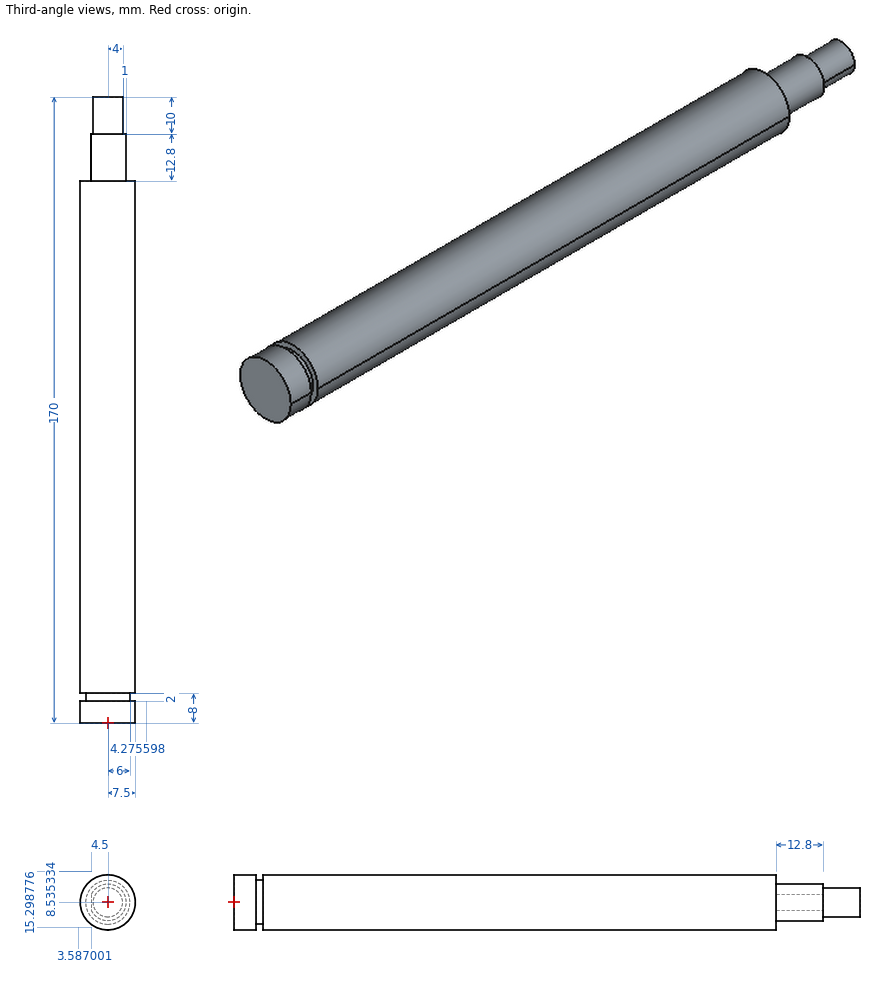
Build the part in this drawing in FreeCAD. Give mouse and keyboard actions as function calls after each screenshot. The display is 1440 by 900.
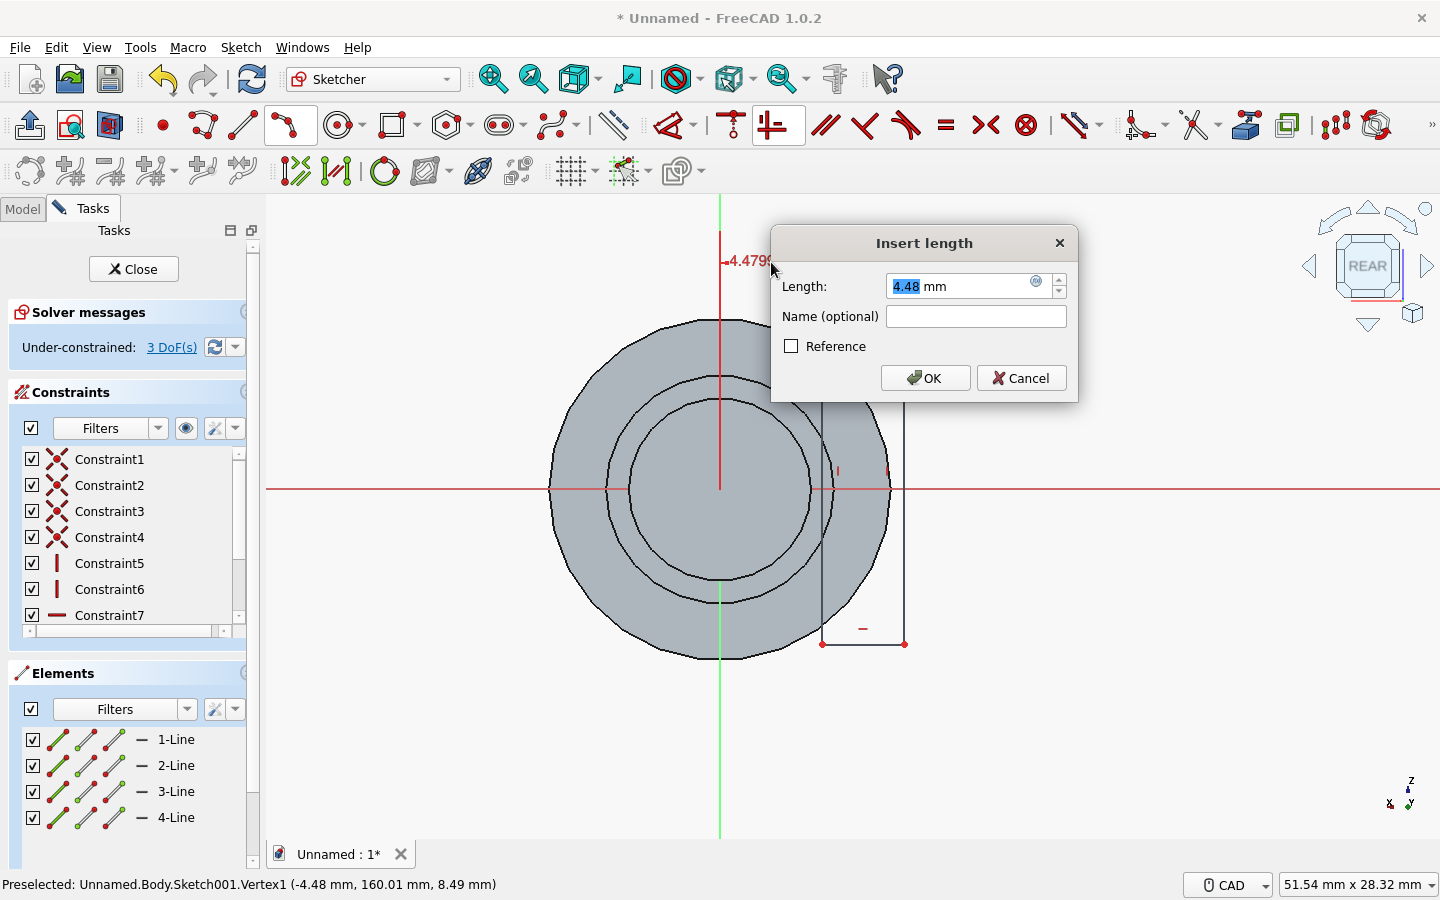
text(4.5)
key(Return)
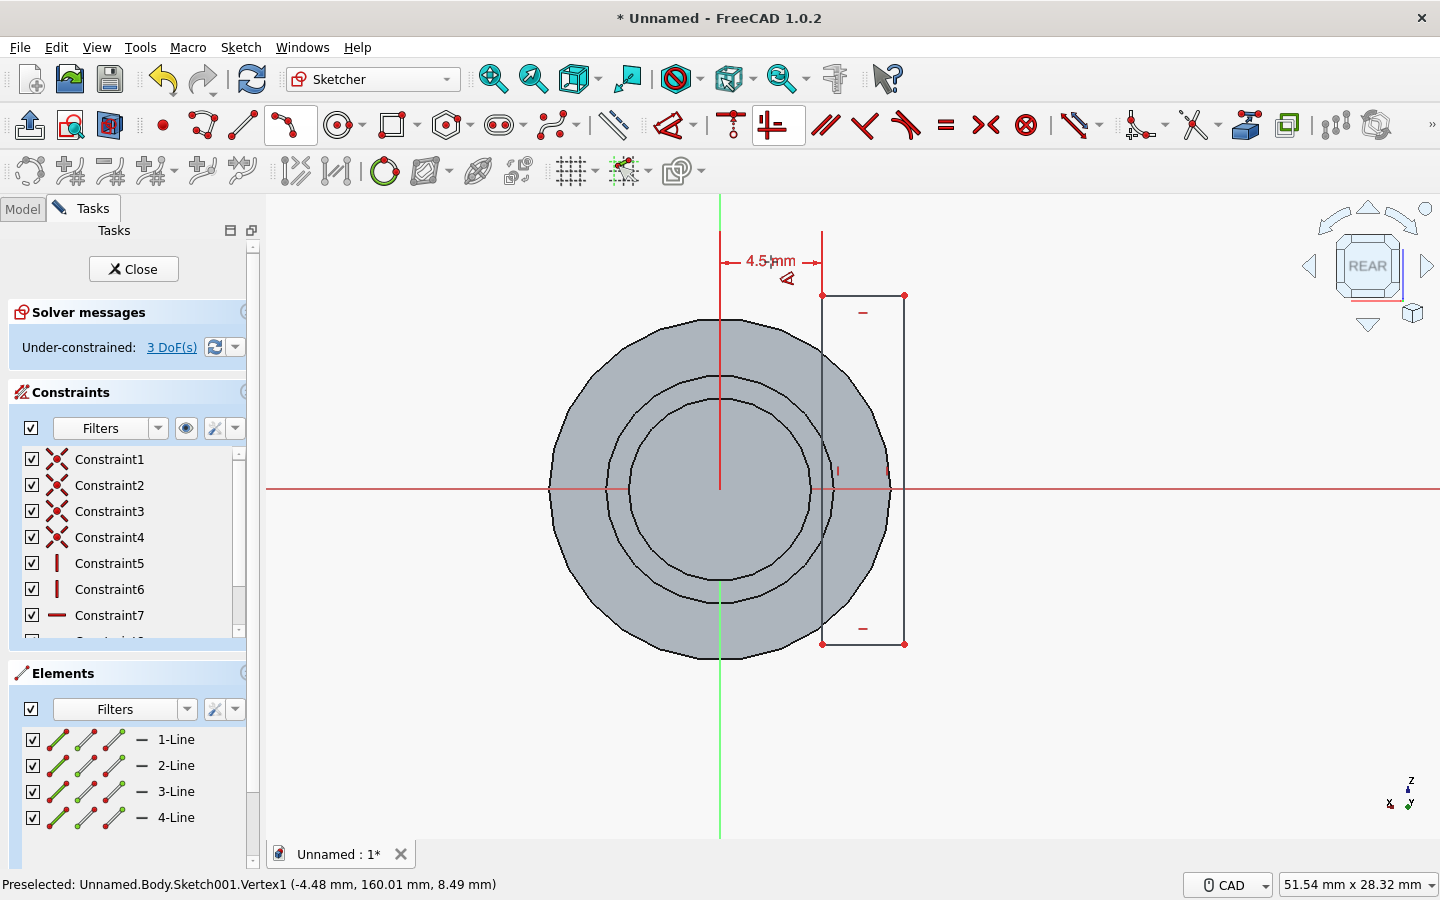
click(847, 645)
click(863, 679)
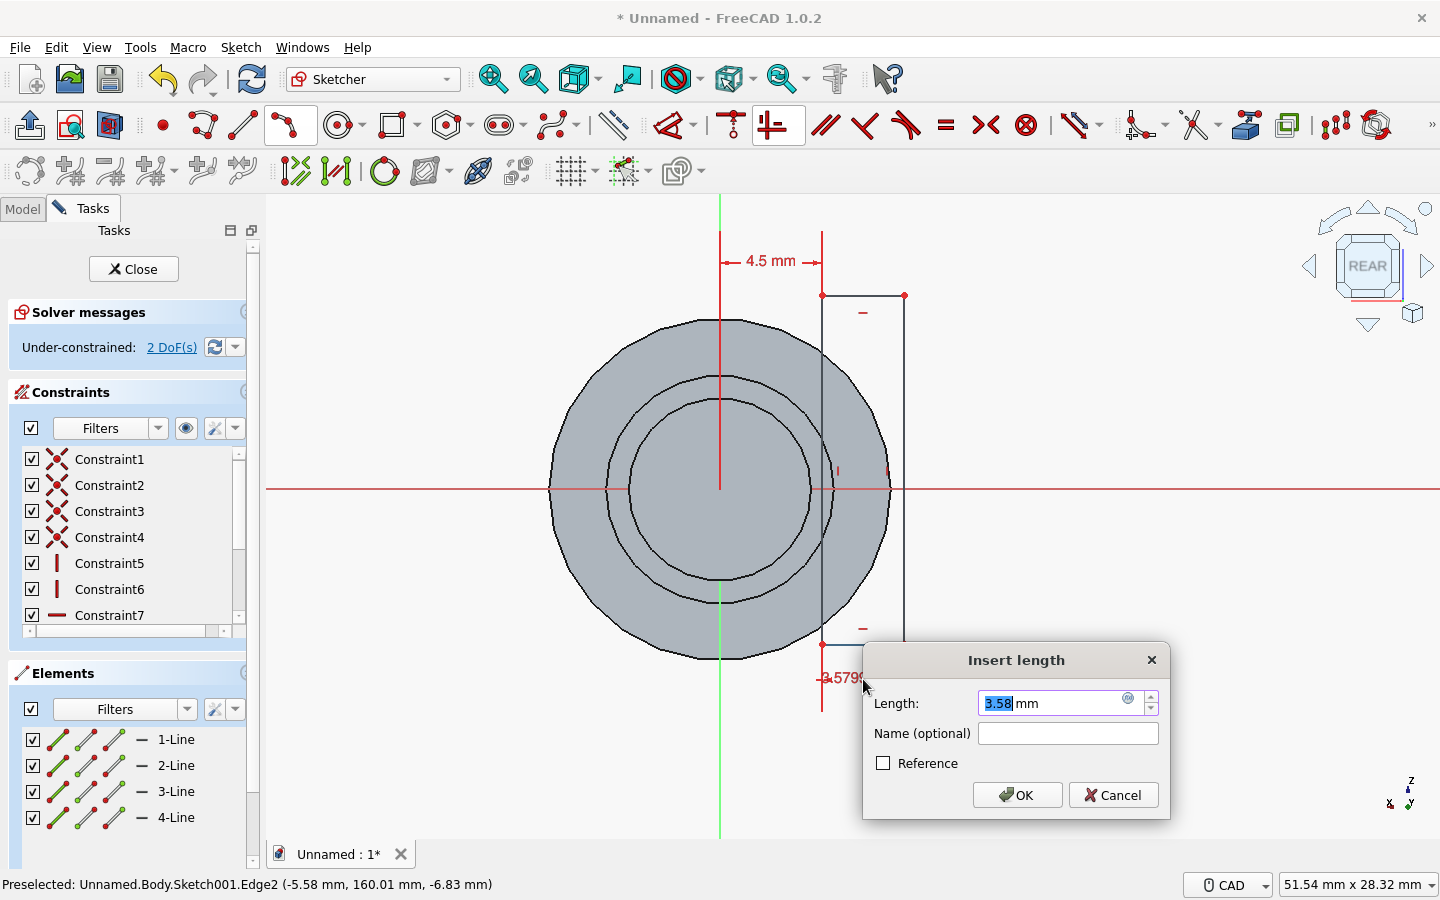
text(3.587001)
key(Return)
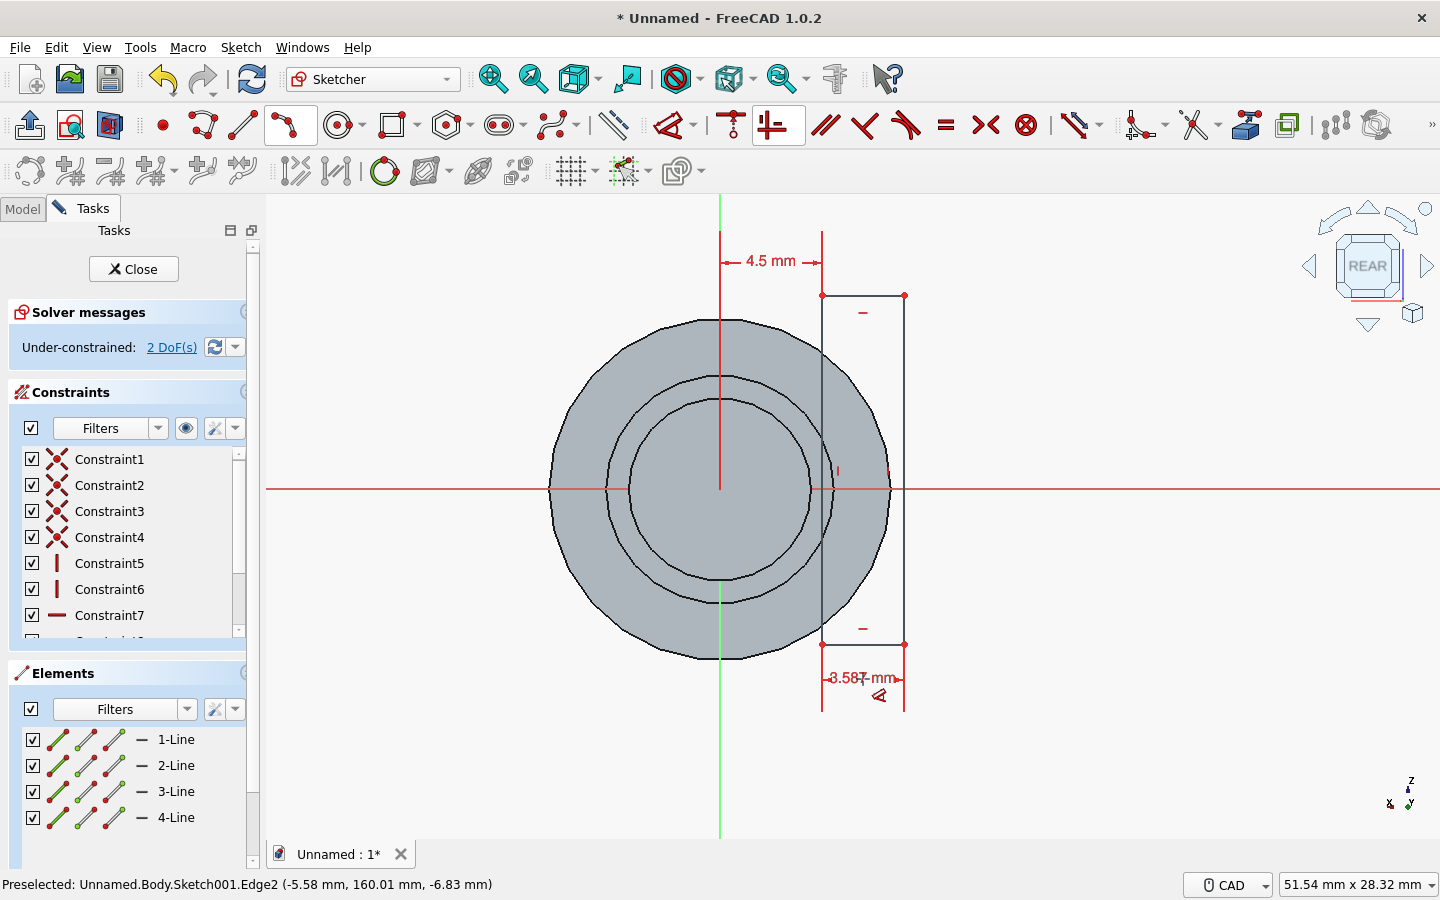
click(822, 401)
click(856, 470)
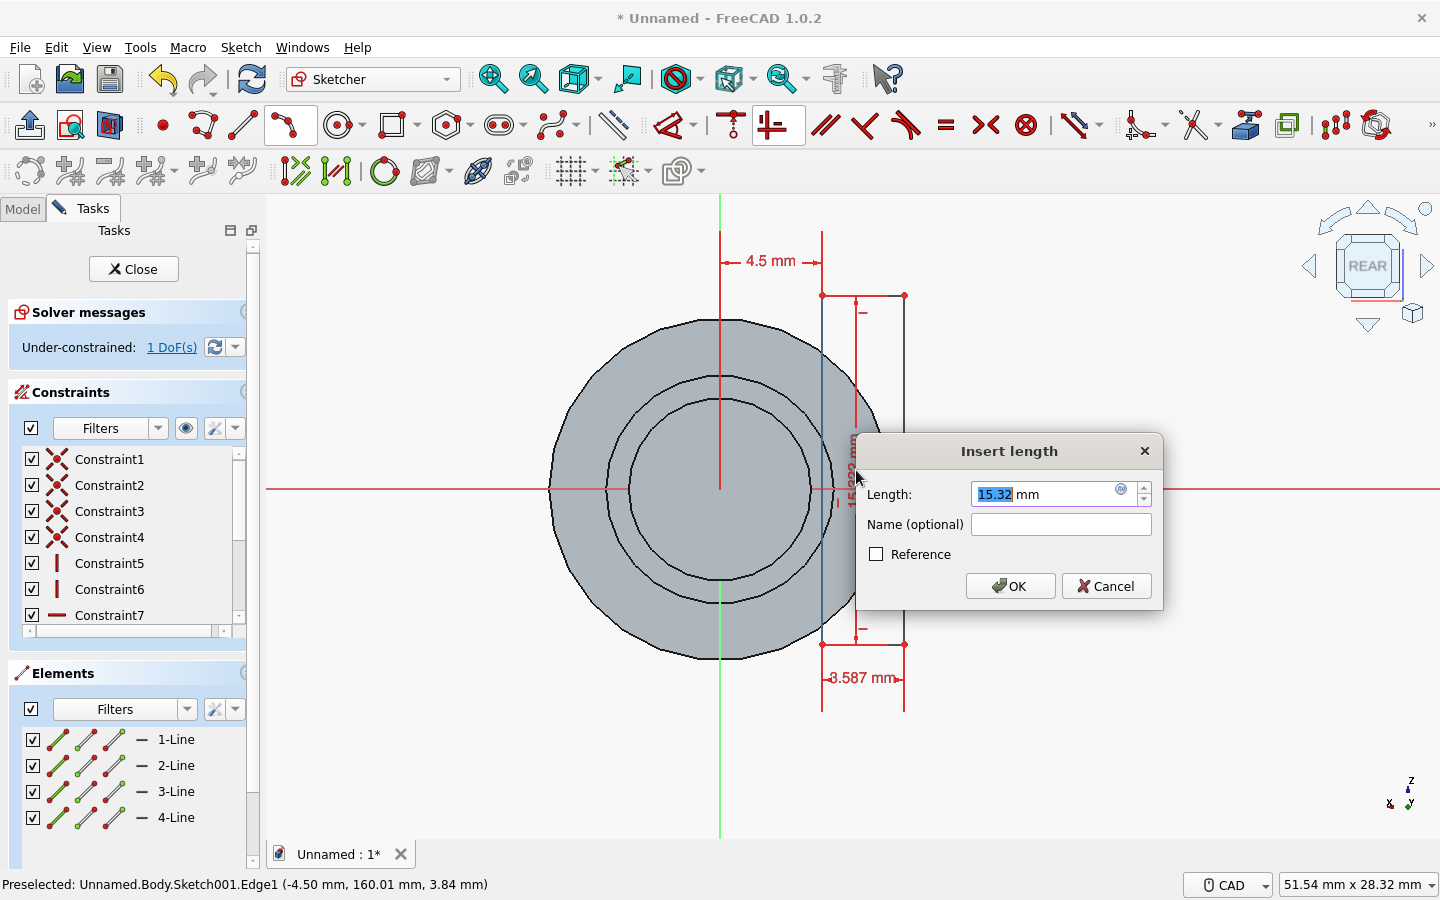
text(15.298776)
key(Return)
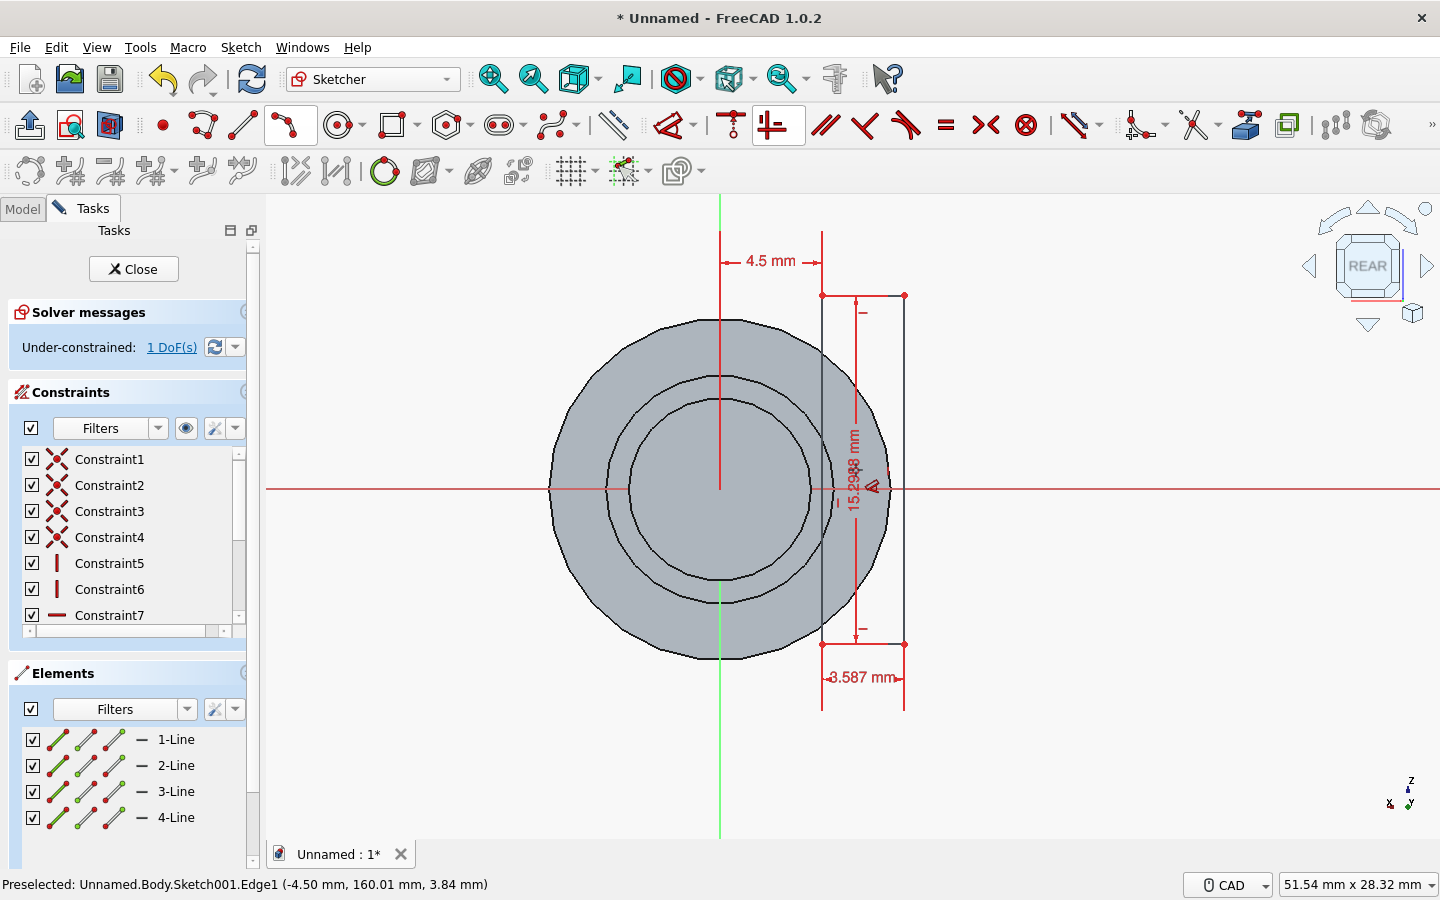
click(822, 296)
click(686, 393)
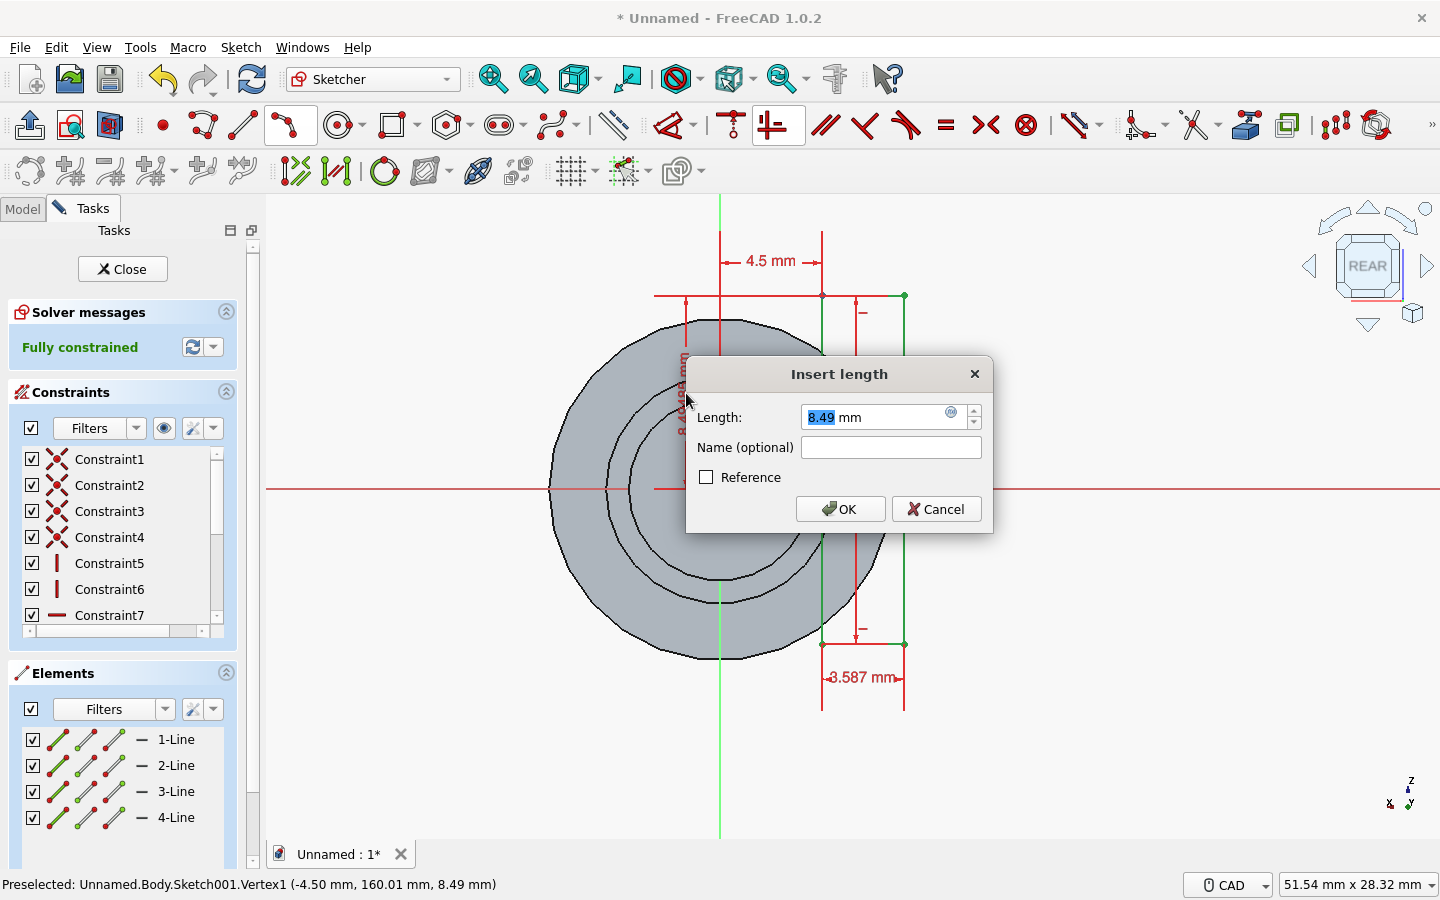
text(8.535334)
key(Return)
key(Escape)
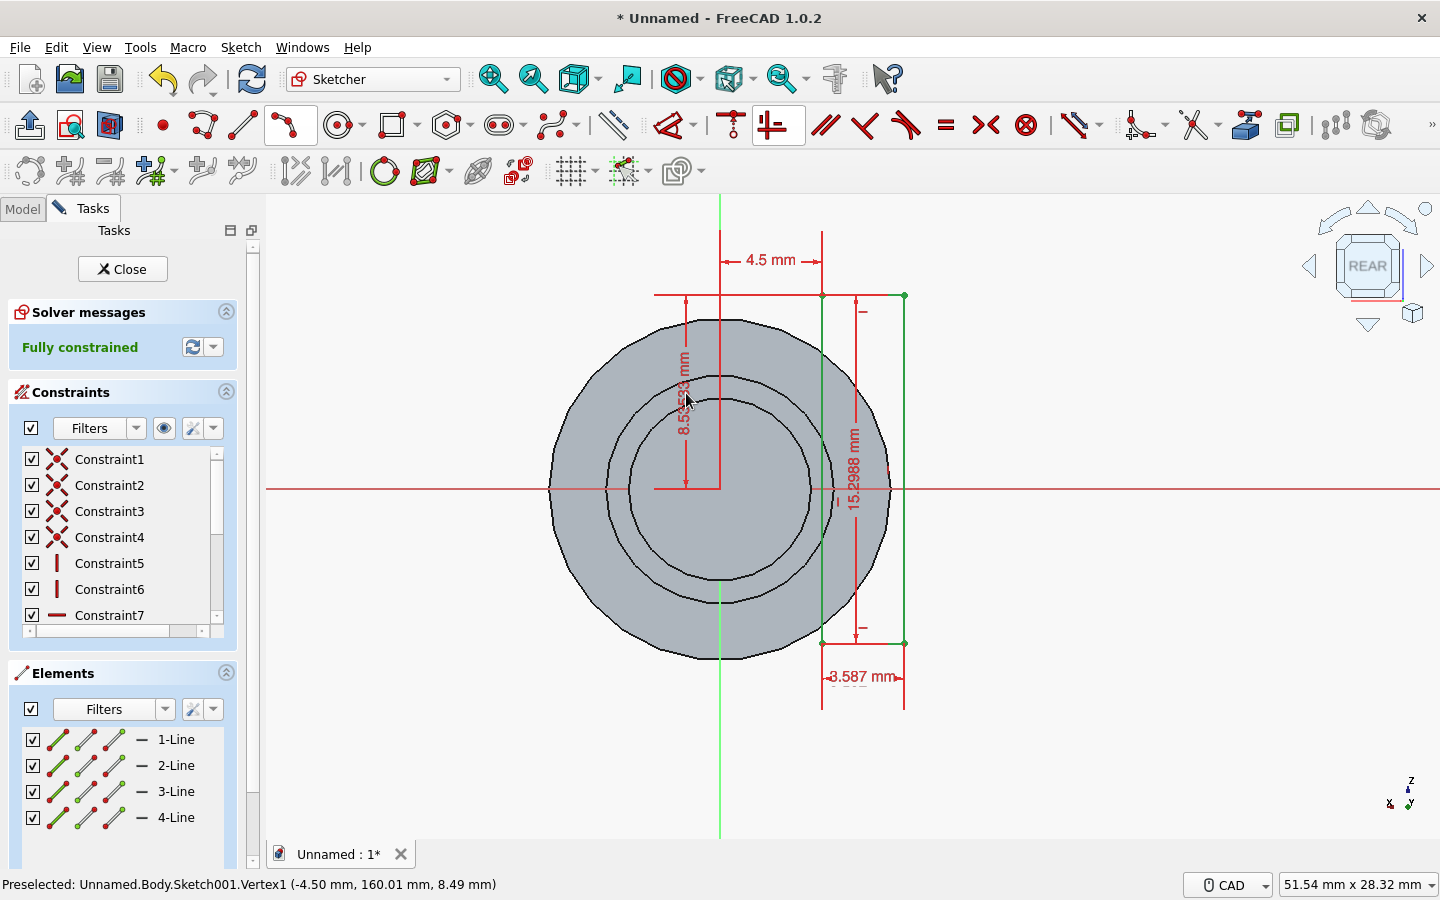
click(123, 269)